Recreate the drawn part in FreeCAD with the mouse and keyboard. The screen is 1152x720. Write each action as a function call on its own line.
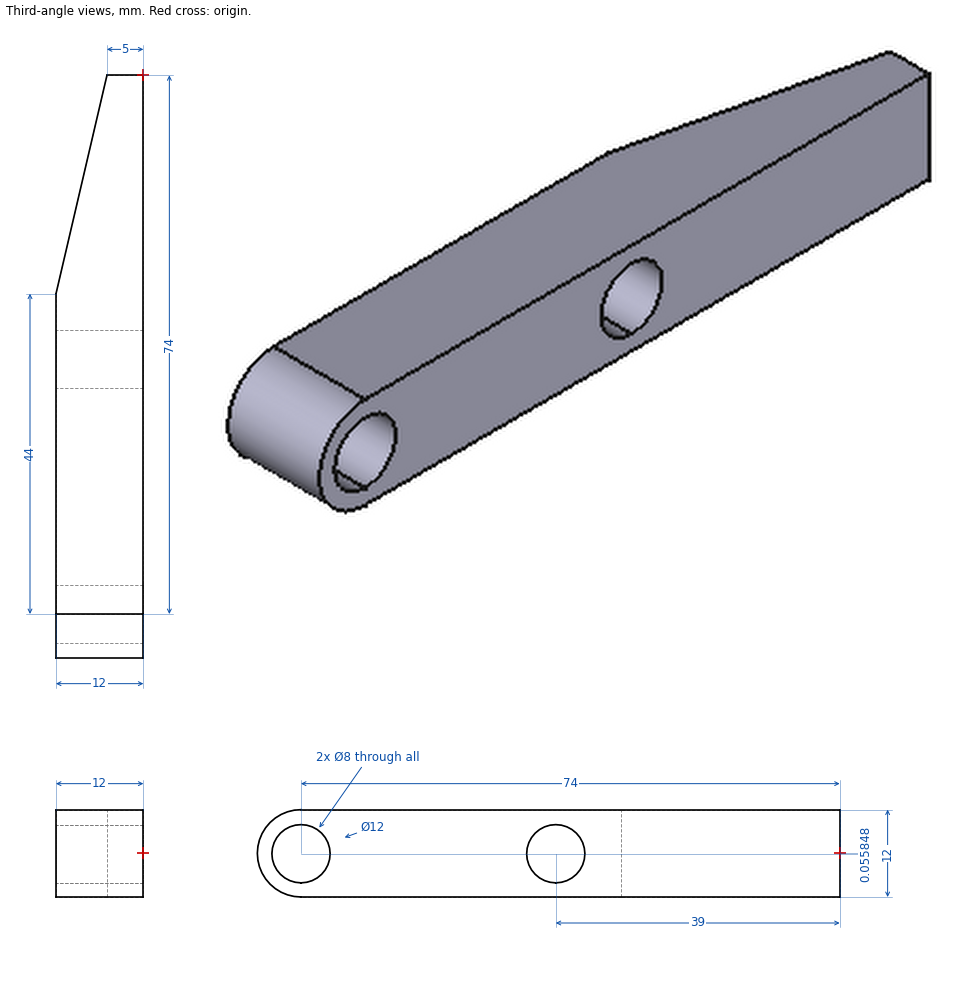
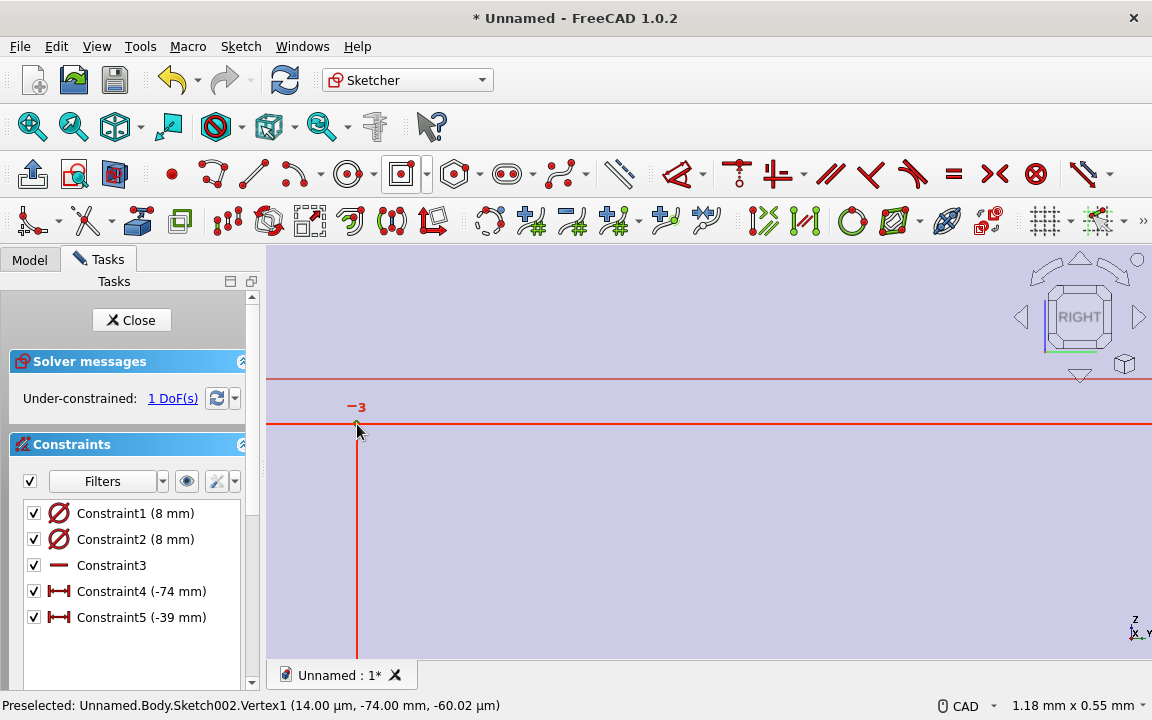
key(i)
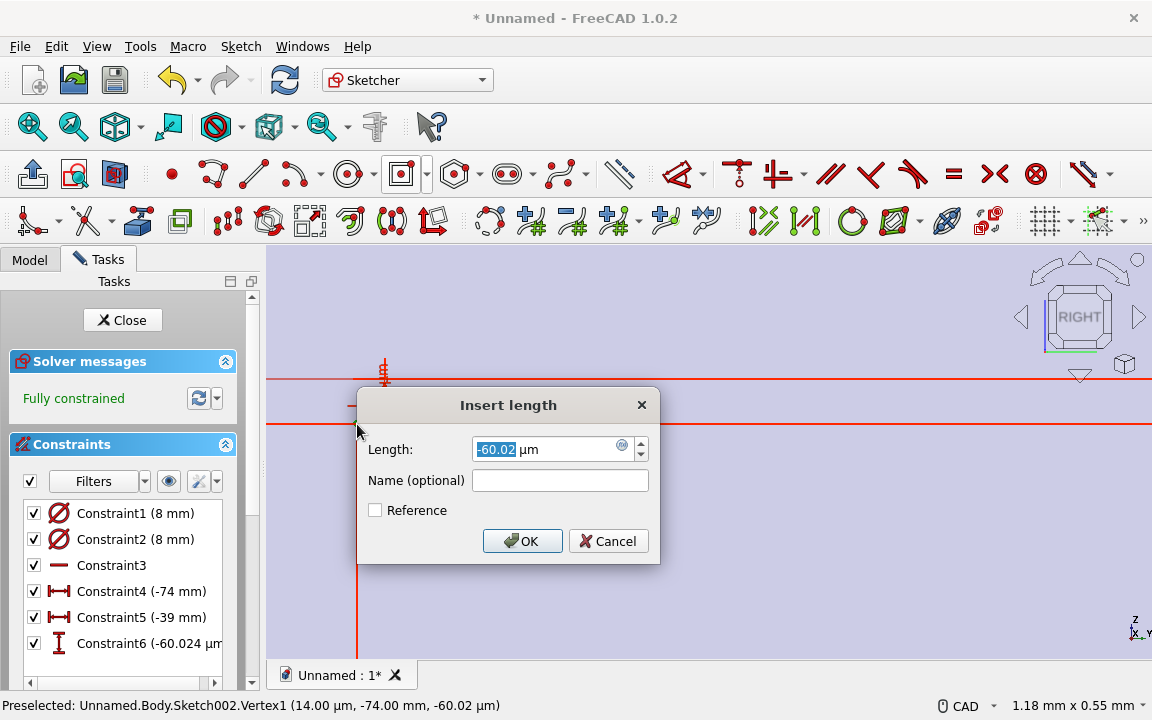
key(ctrl+a)
text(-0.055848 mm)
key(Return)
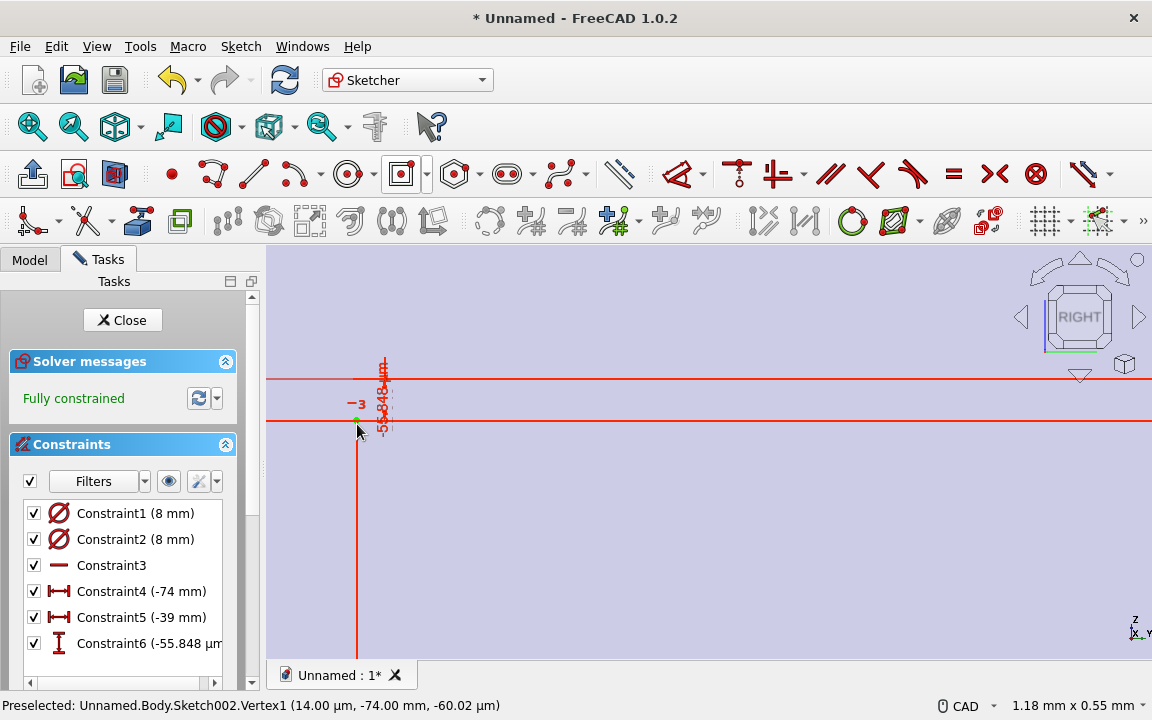
click(123, 320)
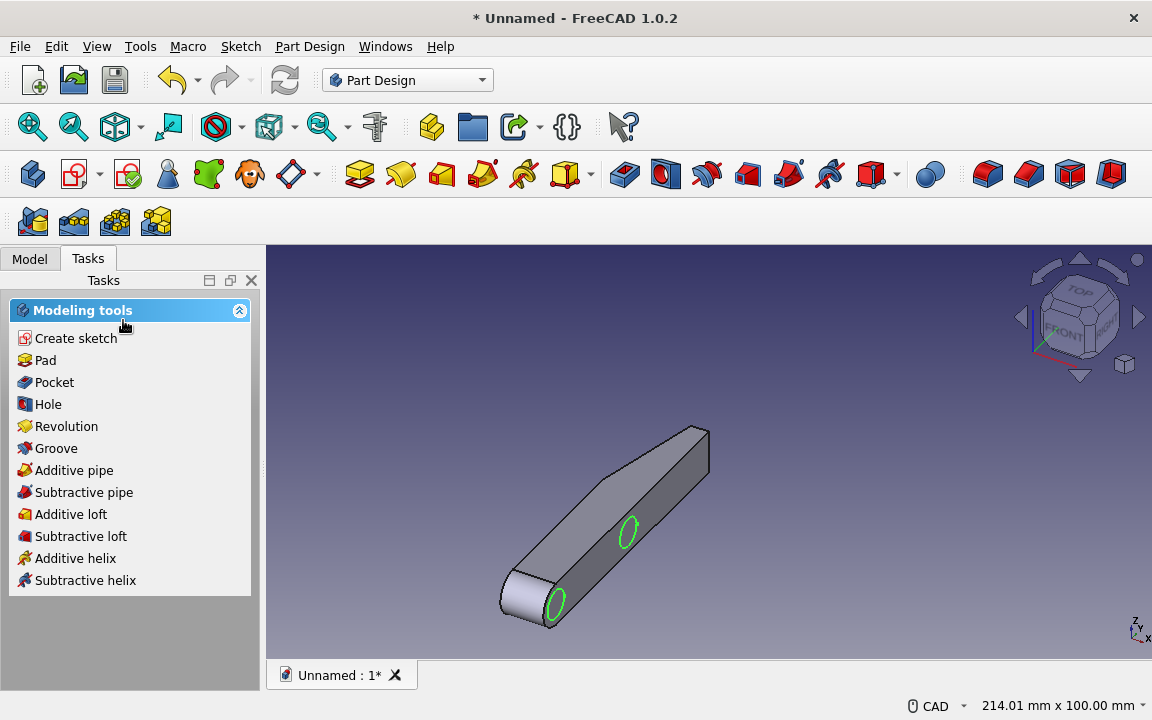
click(666, 174)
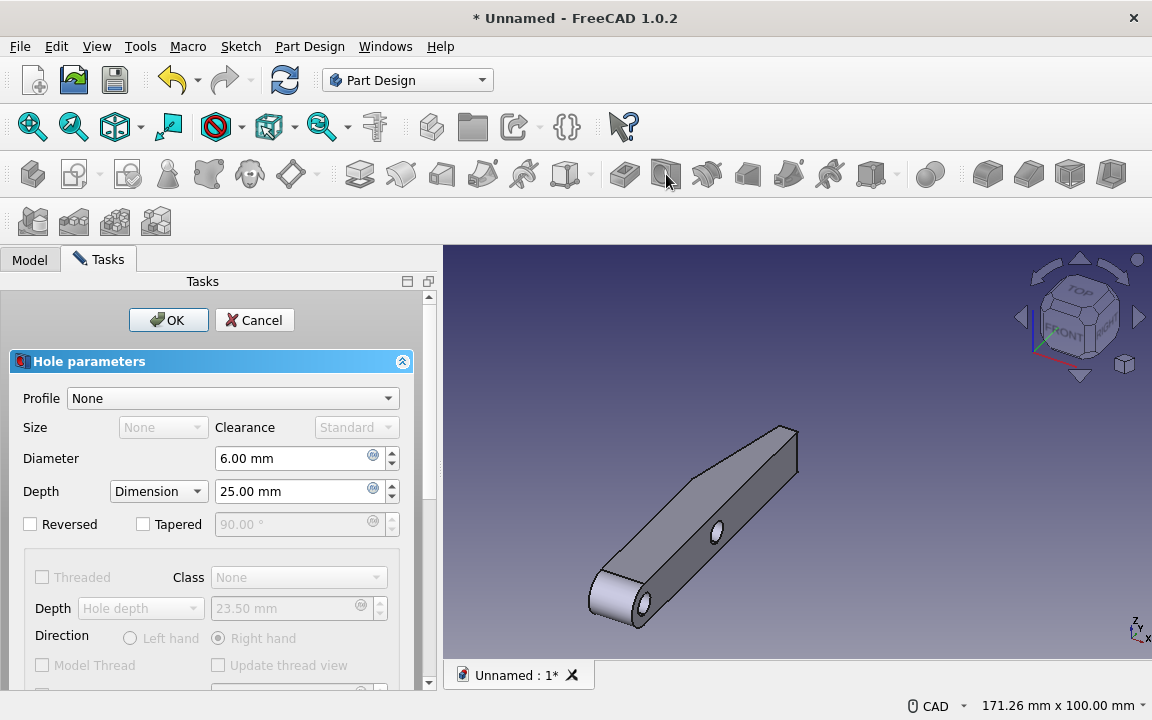
triple_click(300, 458)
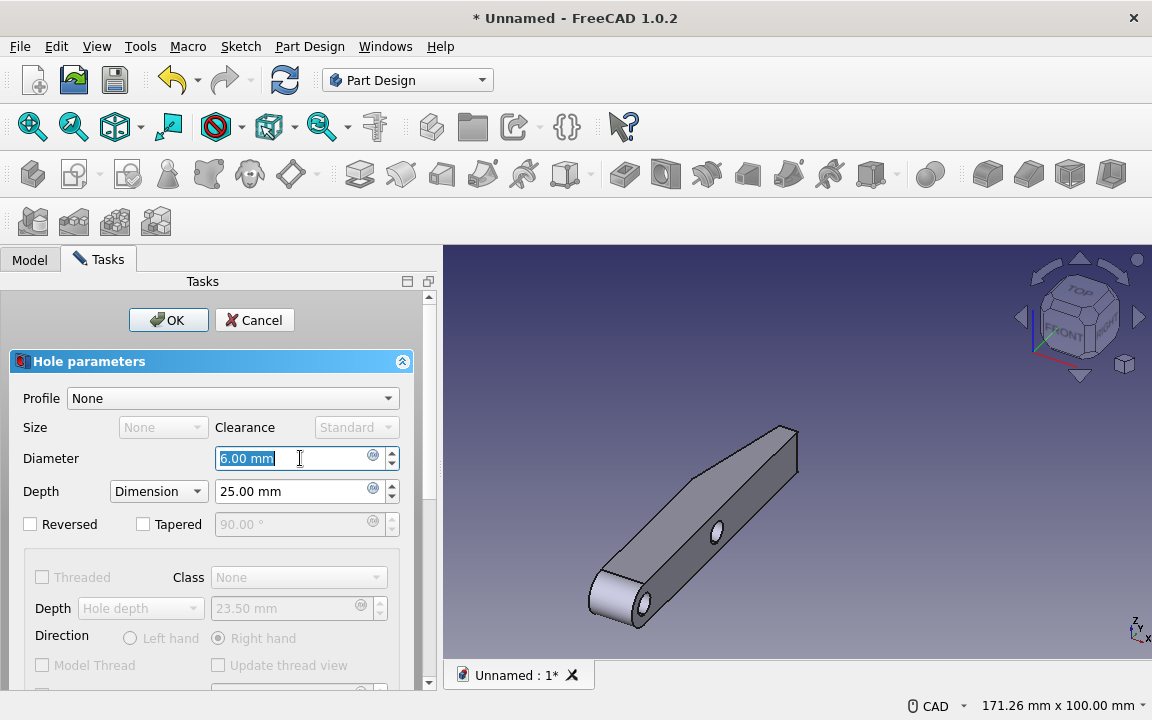
text(8)
key(Tab)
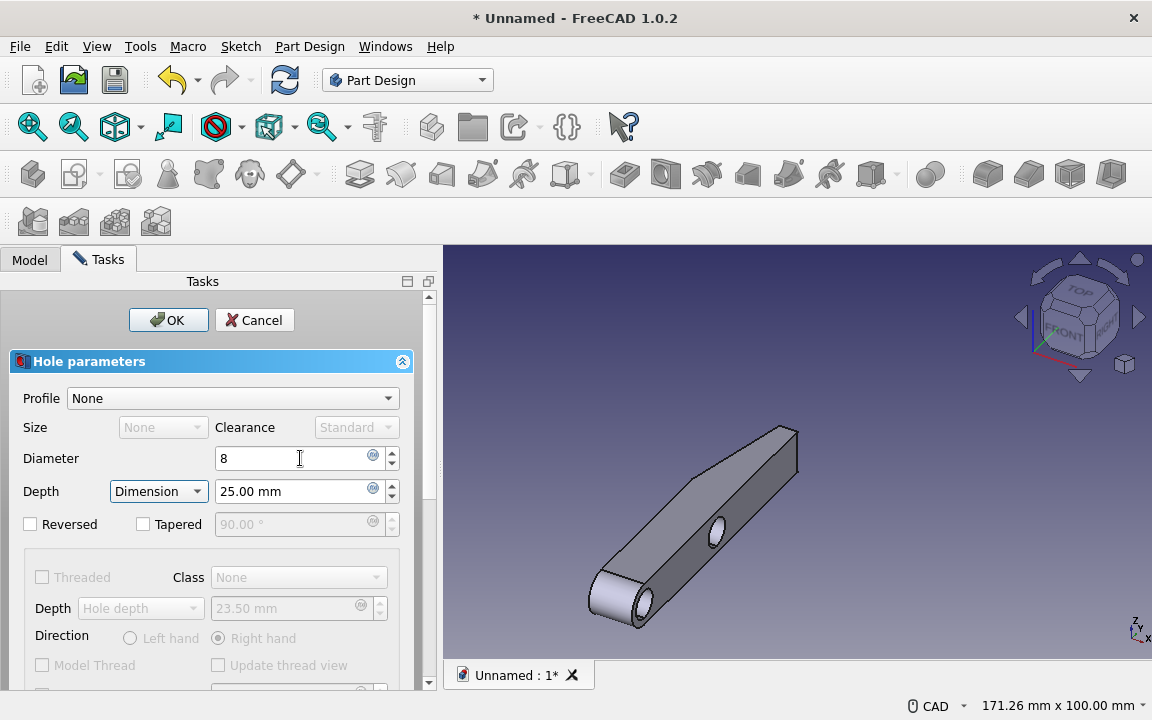
click(160, 492)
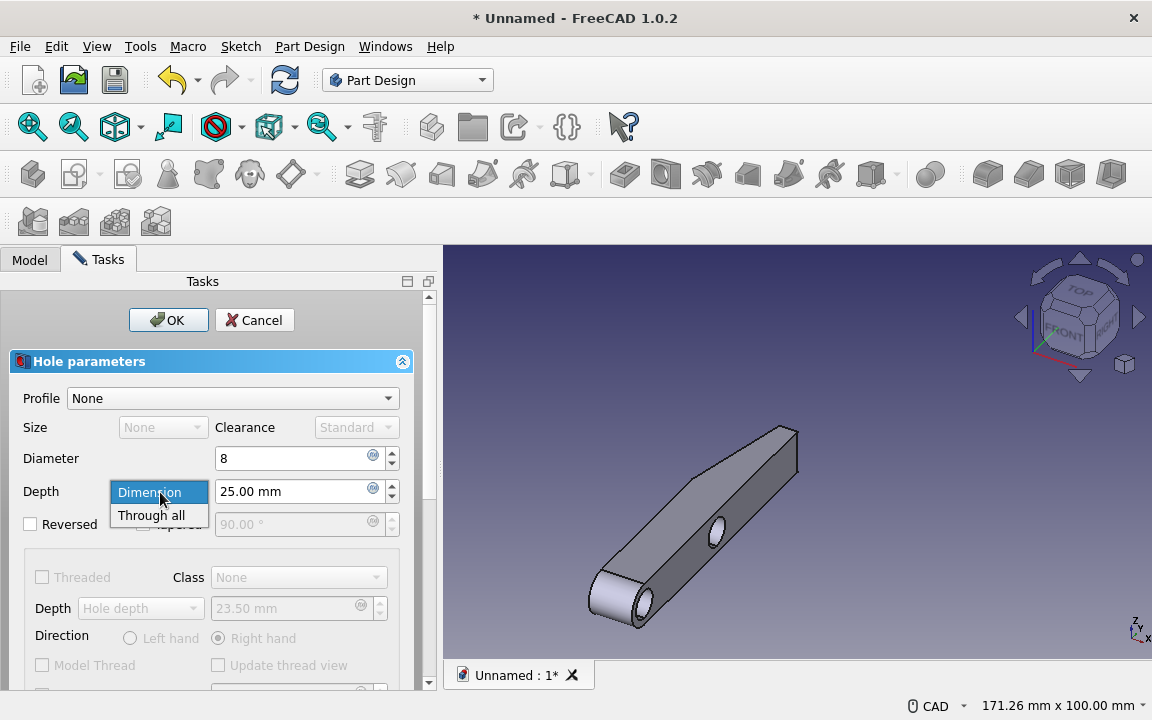
click(158, 516)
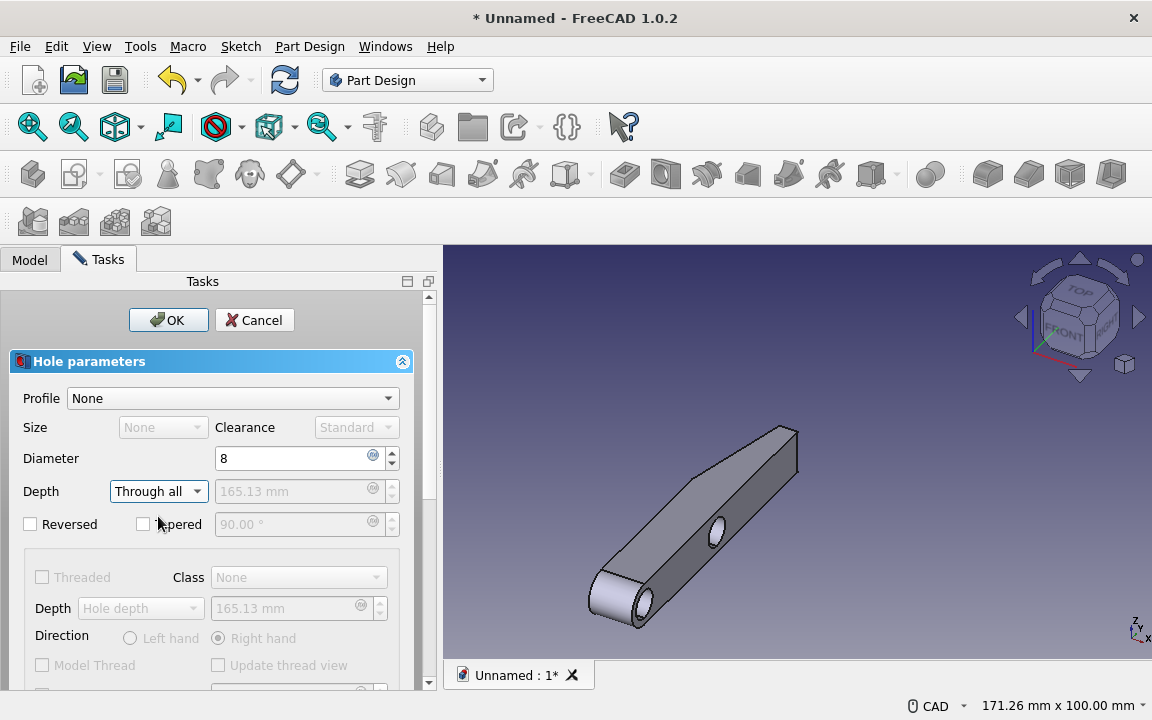
click(169, 320)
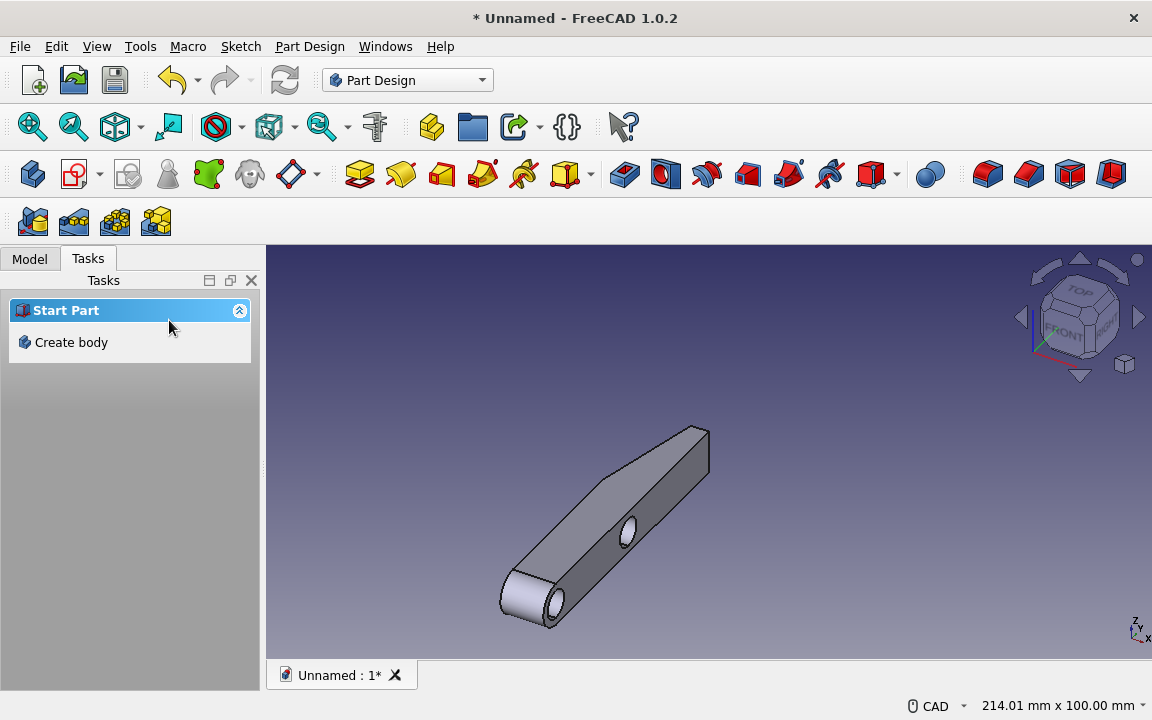
key(0)